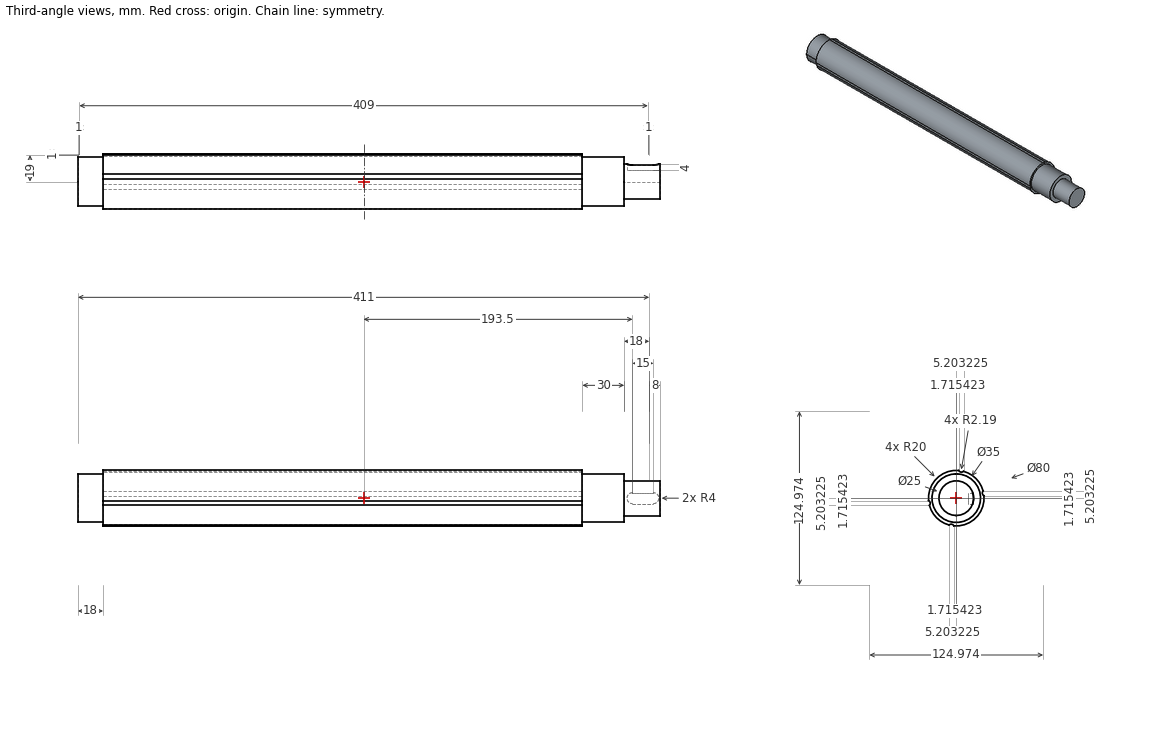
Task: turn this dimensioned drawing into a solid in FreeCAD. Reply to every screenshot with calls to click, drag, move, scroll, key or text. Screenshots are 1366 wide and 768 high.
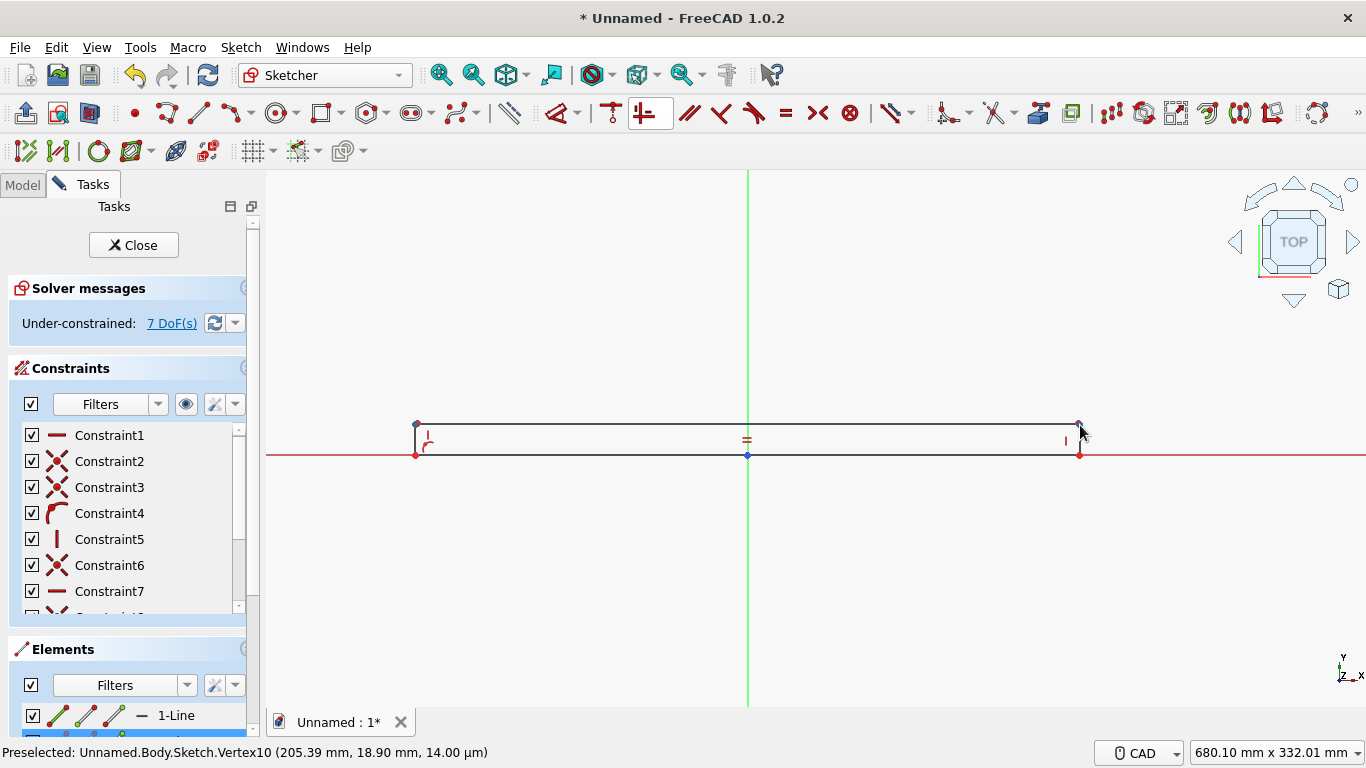
click(748, 645)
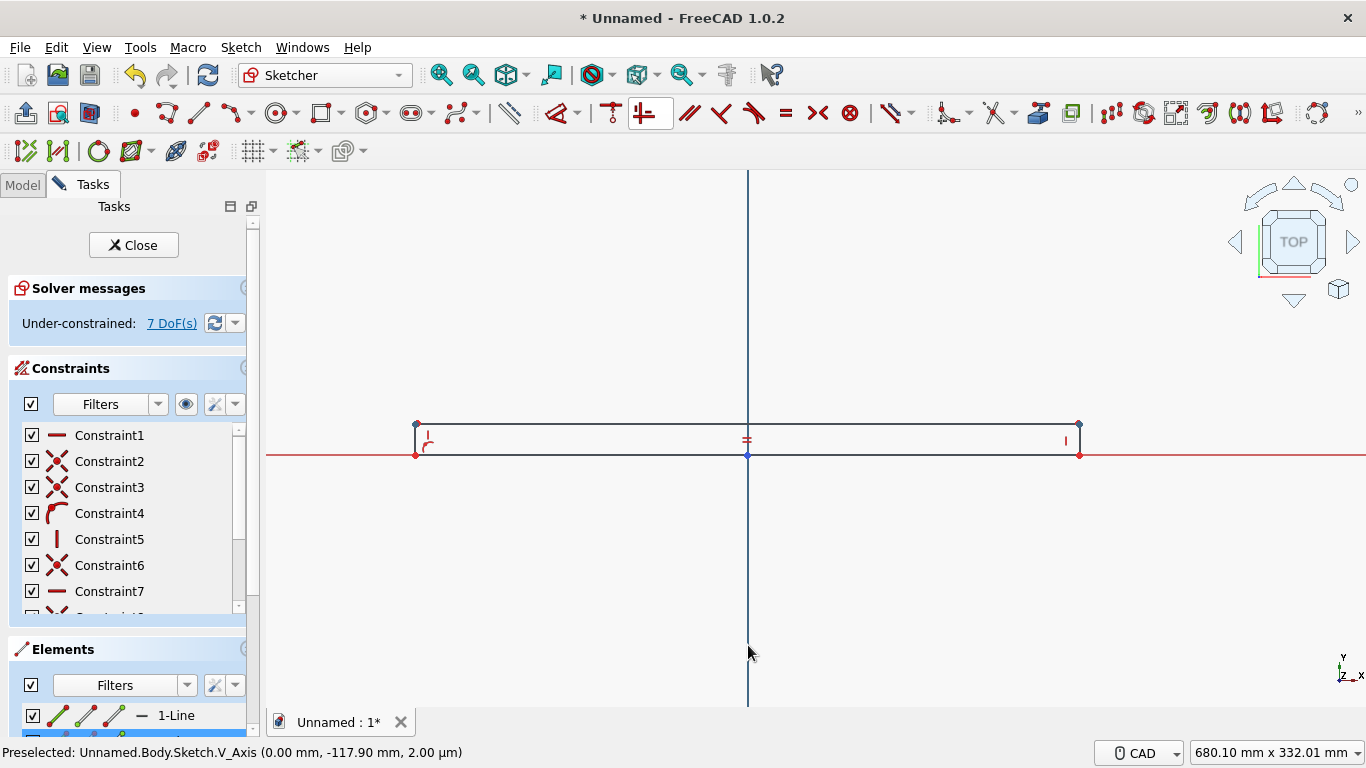
click(818, 114)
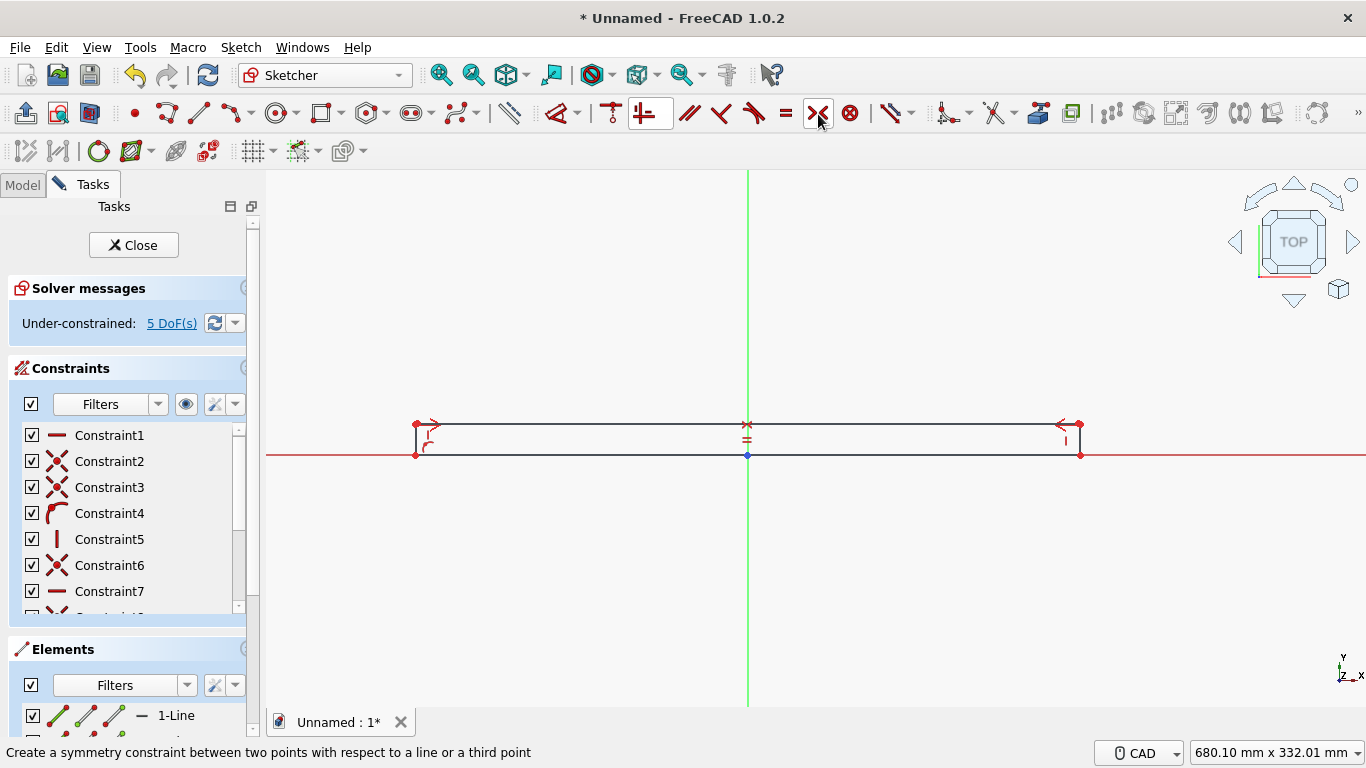
key(d)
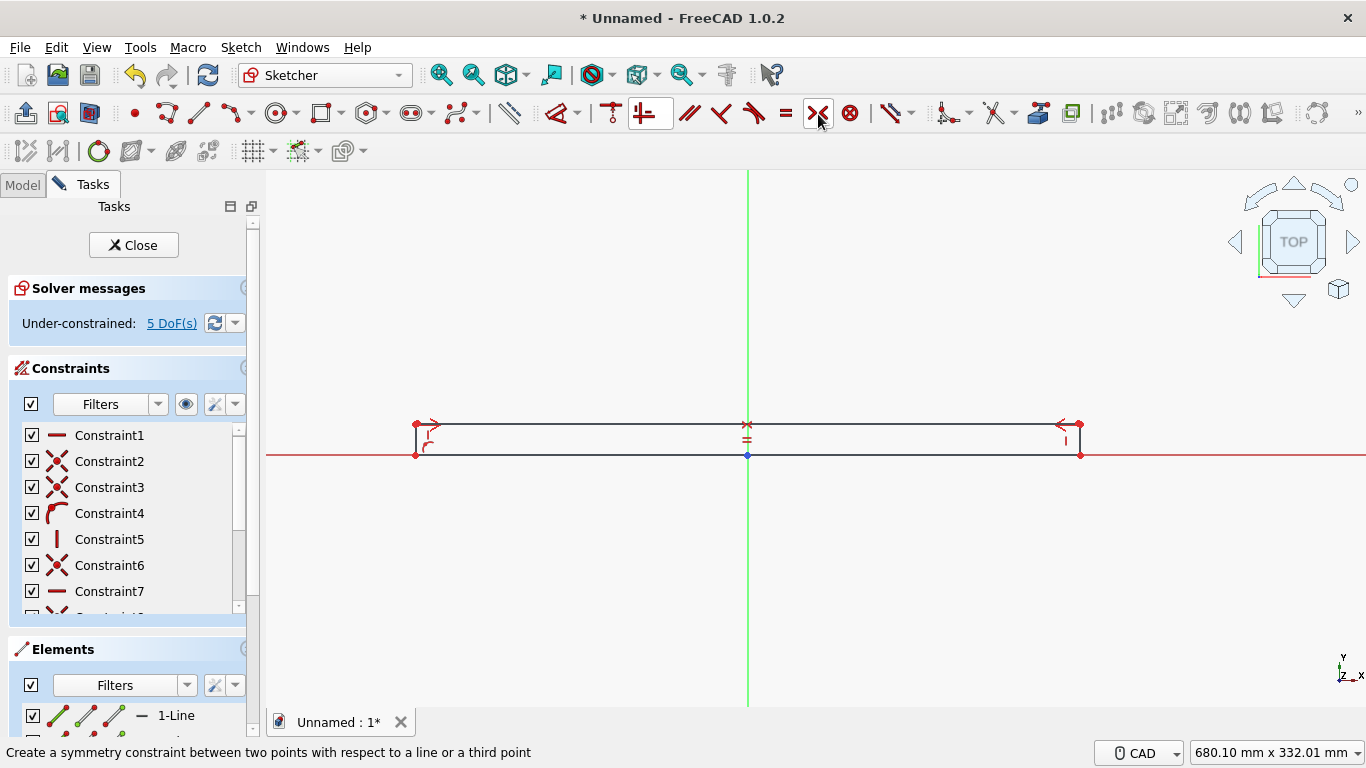
scroll(416, 434, up, 3)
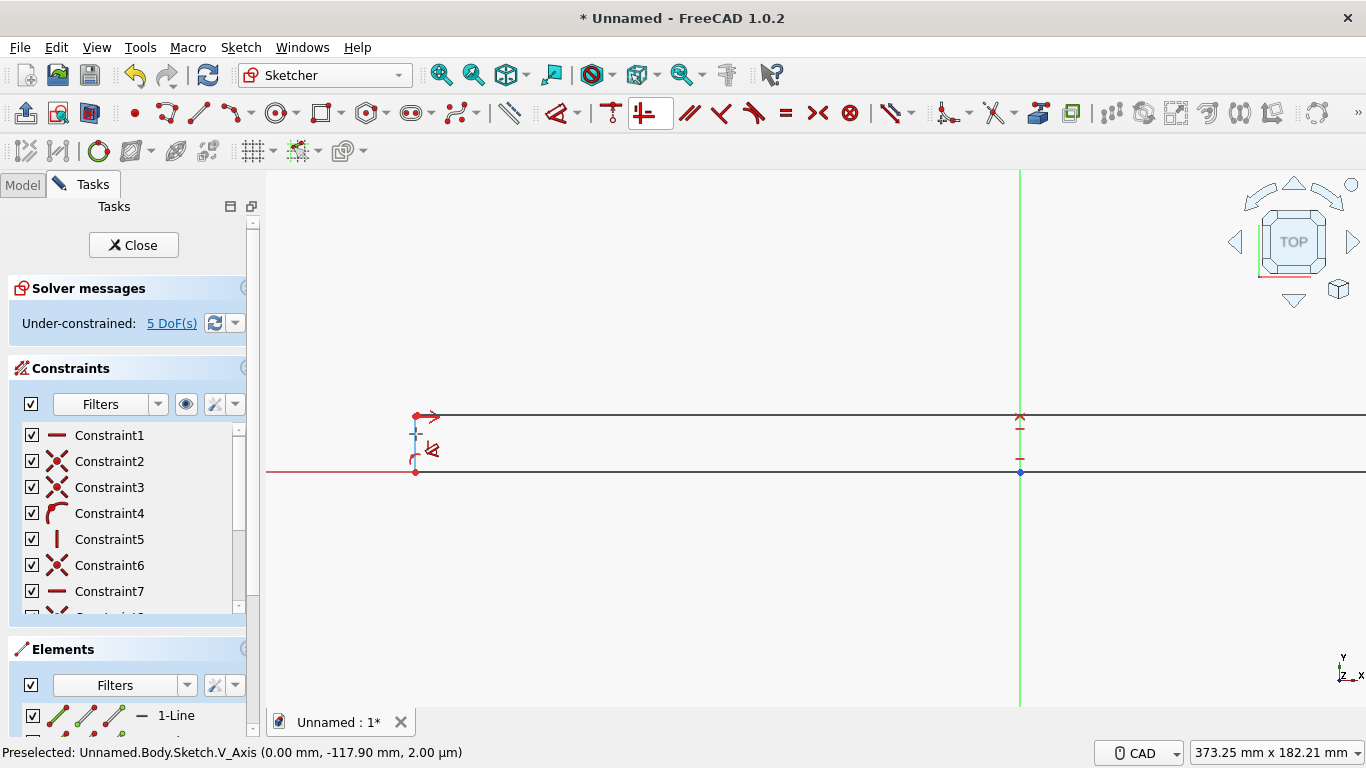
click(415, 433)
click(381, 445)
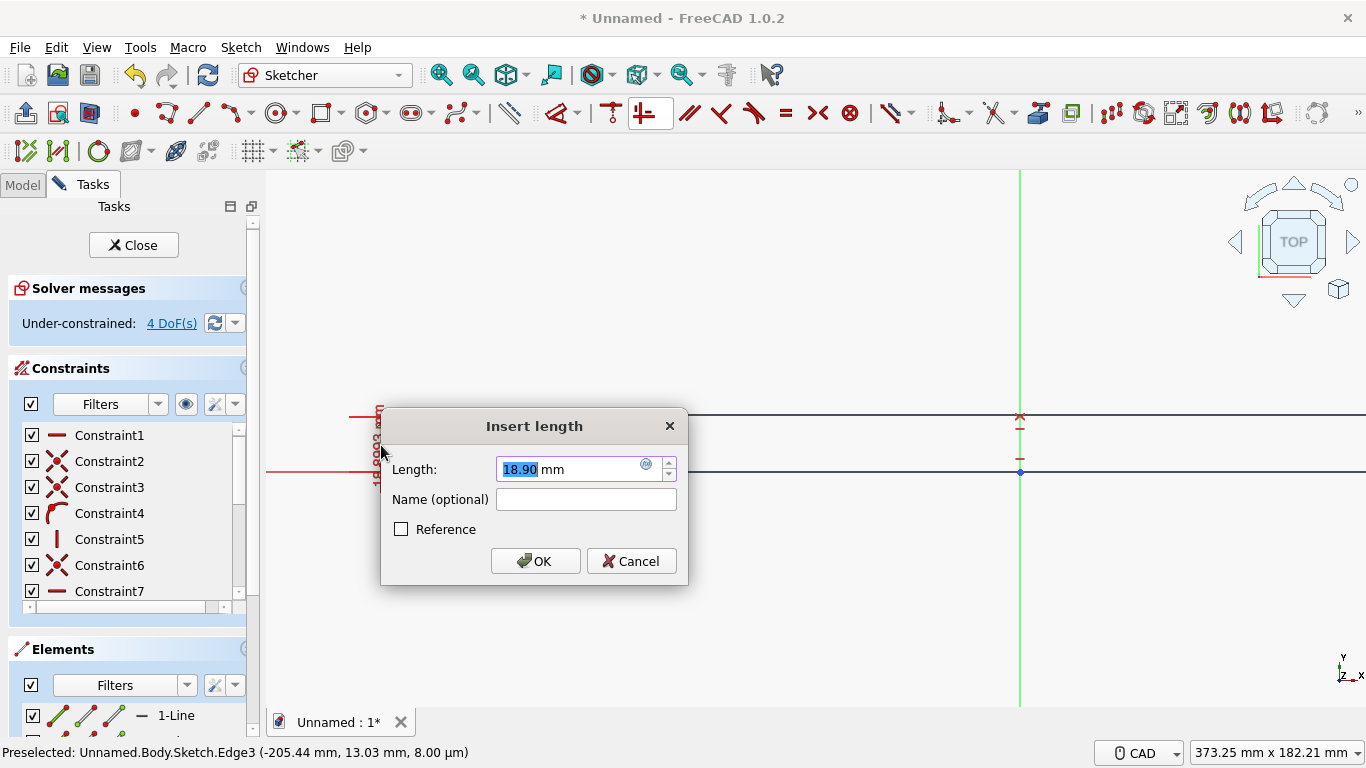
text(19)
key(Return)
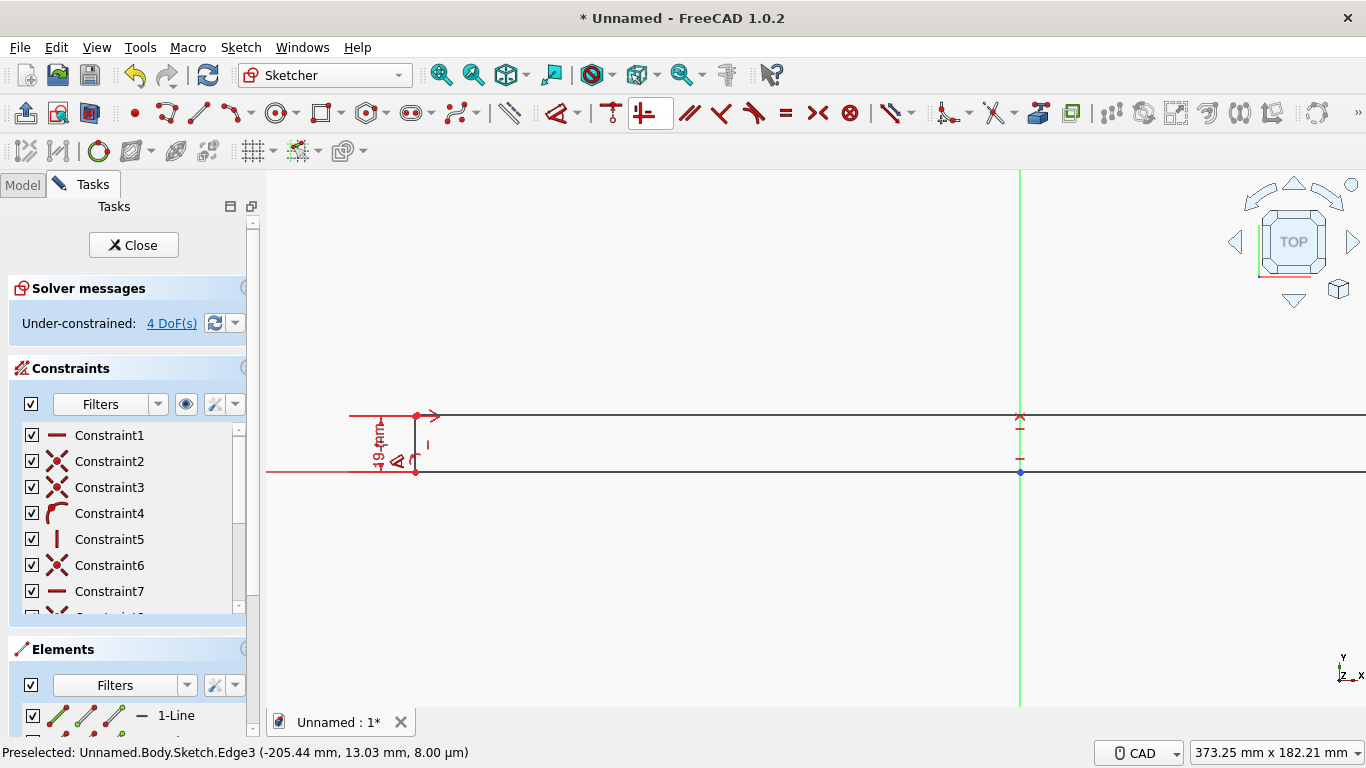
scroll(416, 416, up, 14)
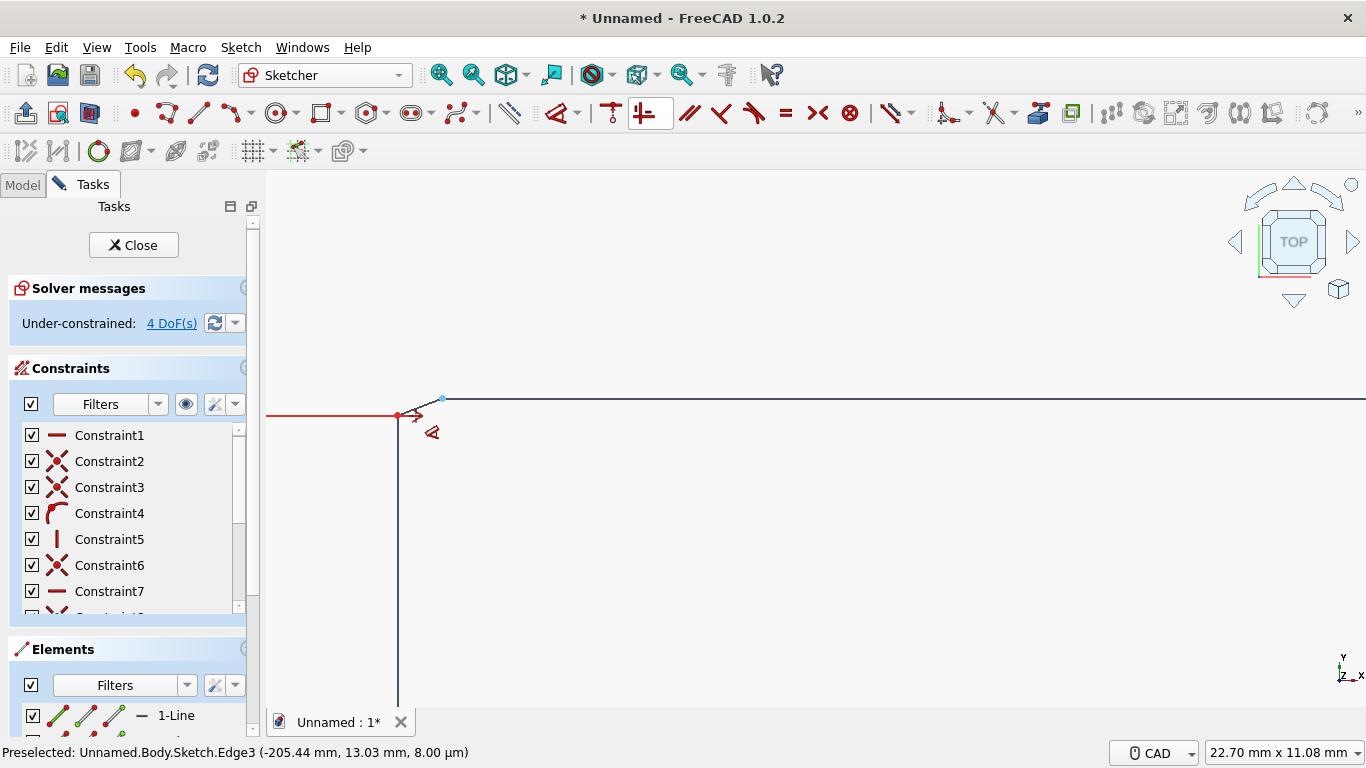
click(420, 407)
click(420, 365)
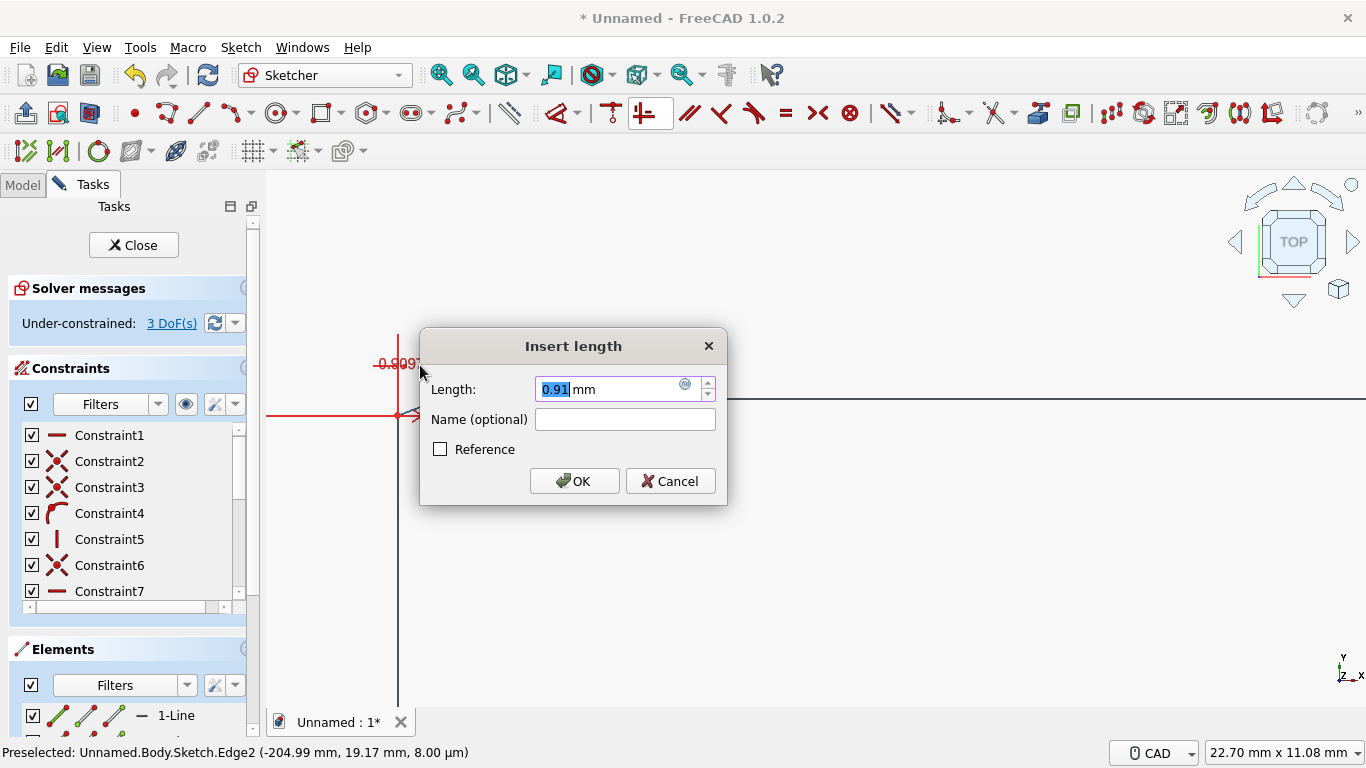
text(1)
key(Return)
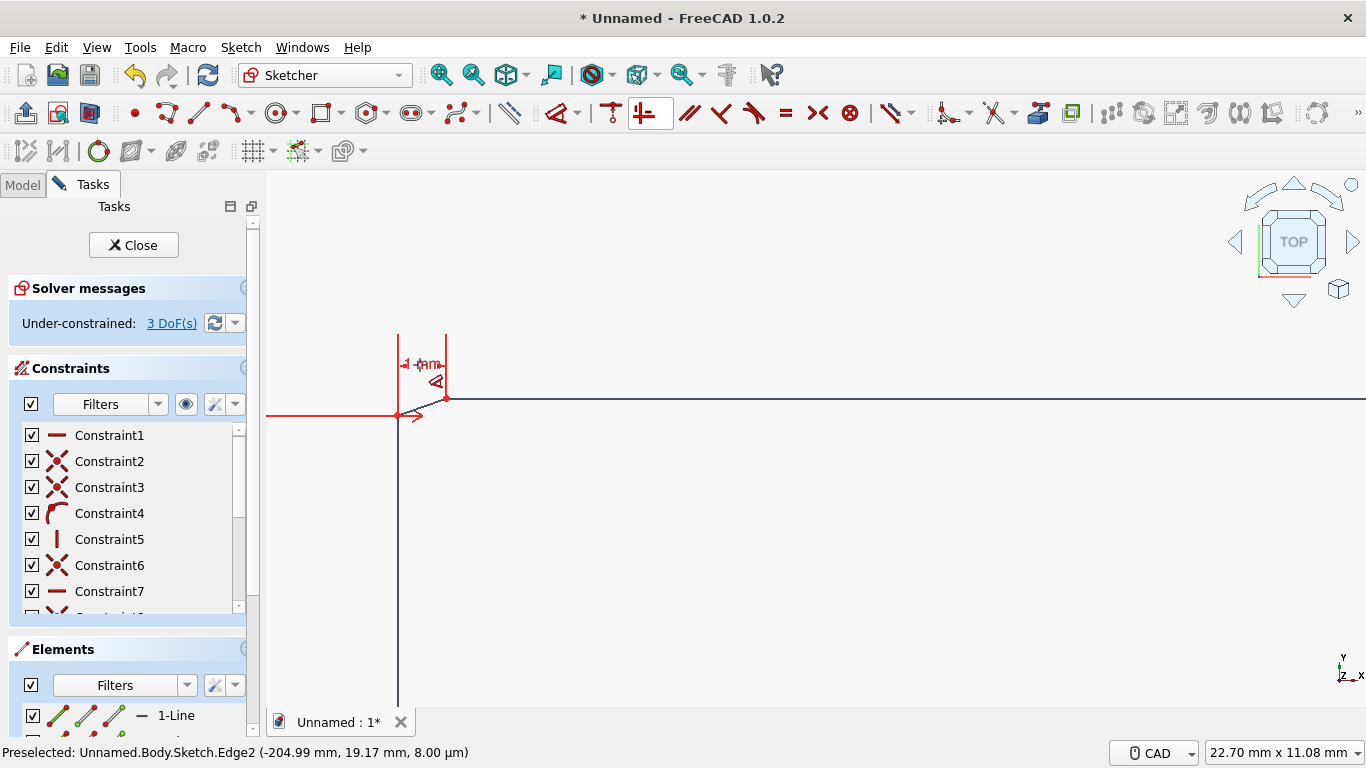
click(432, 404)
click(364, 407)